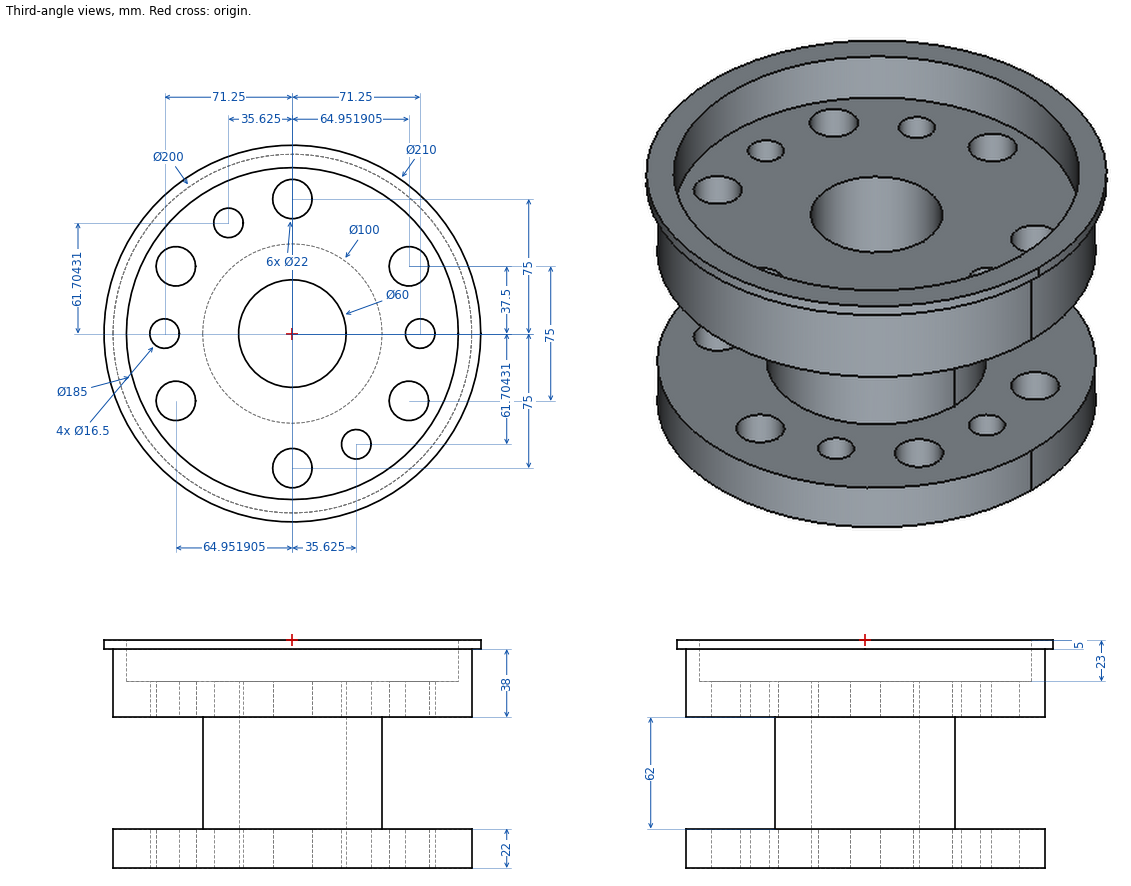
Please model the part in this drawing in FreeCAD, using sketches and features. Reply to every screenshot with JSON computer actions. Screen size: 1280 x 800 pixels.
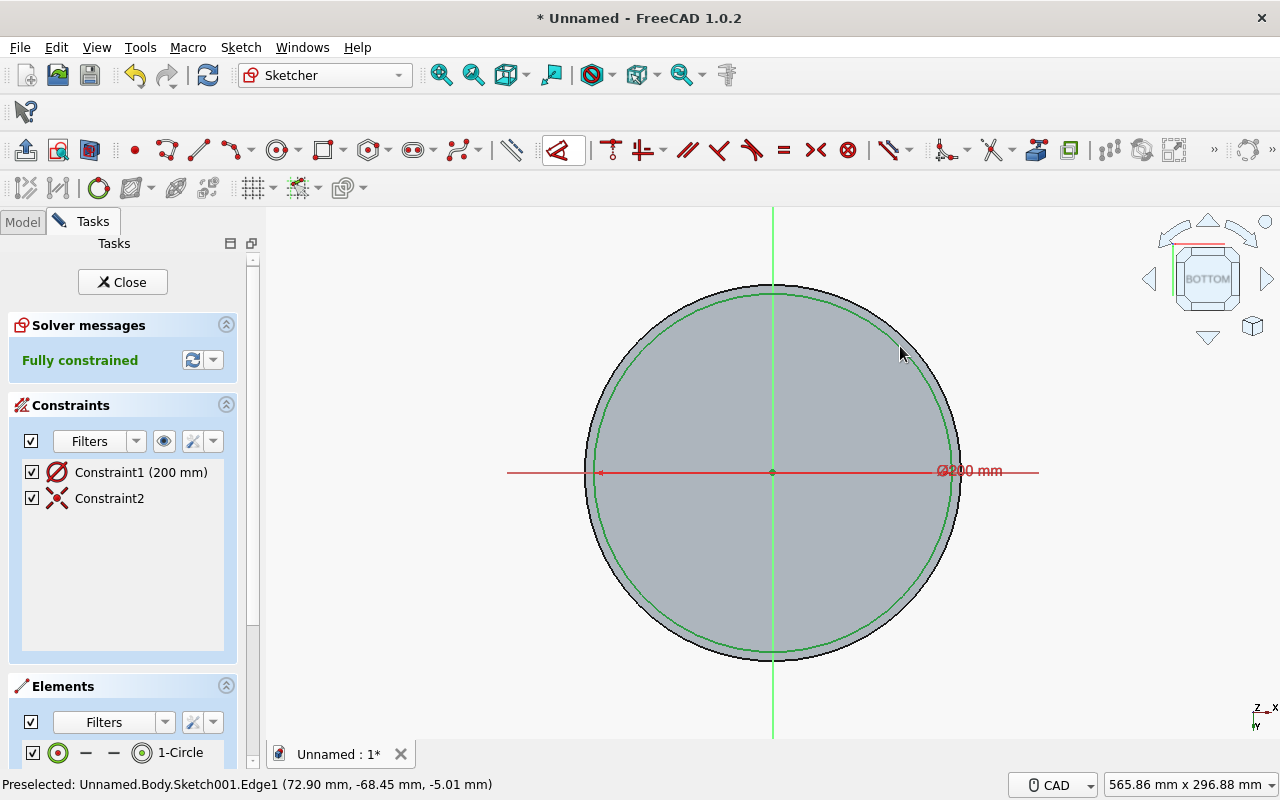
{"action": "left_click", "coordinate": [123, 282]}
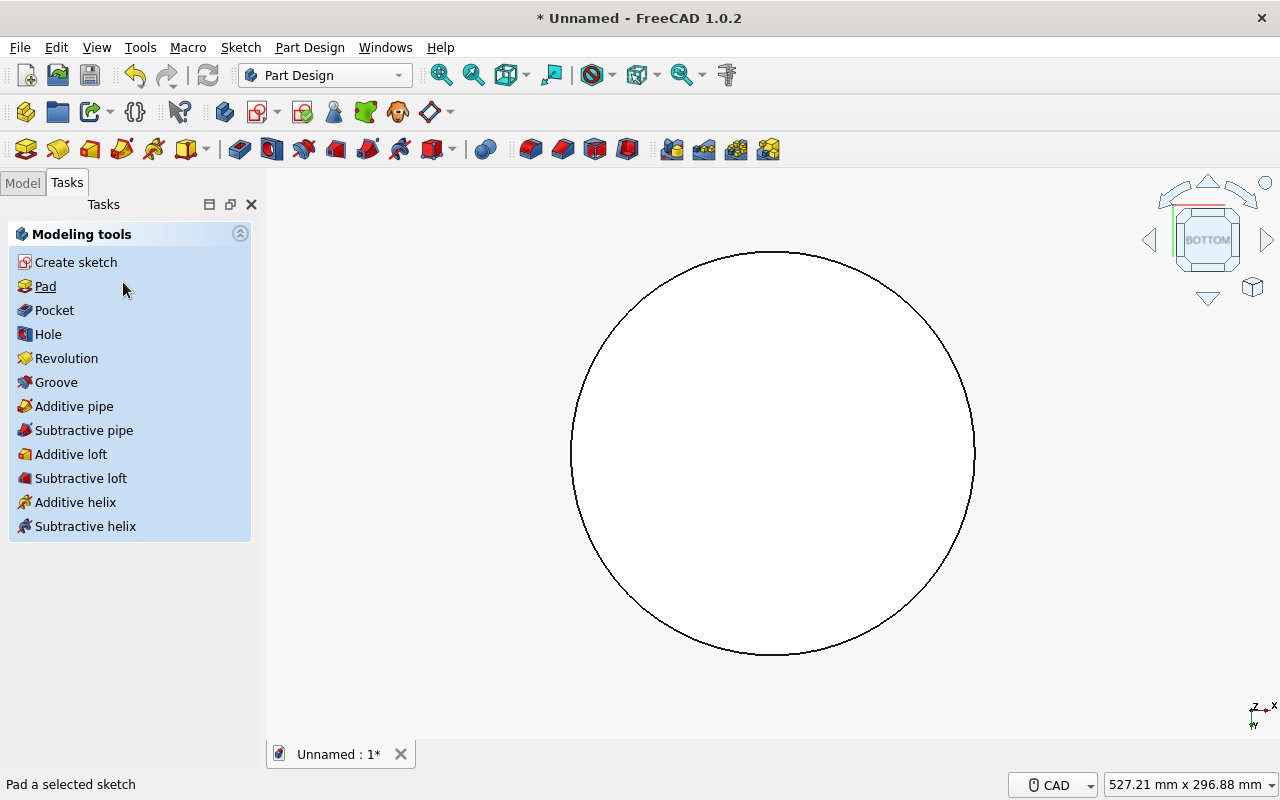
{"action": "left_click", "coordinate": [26, 150]}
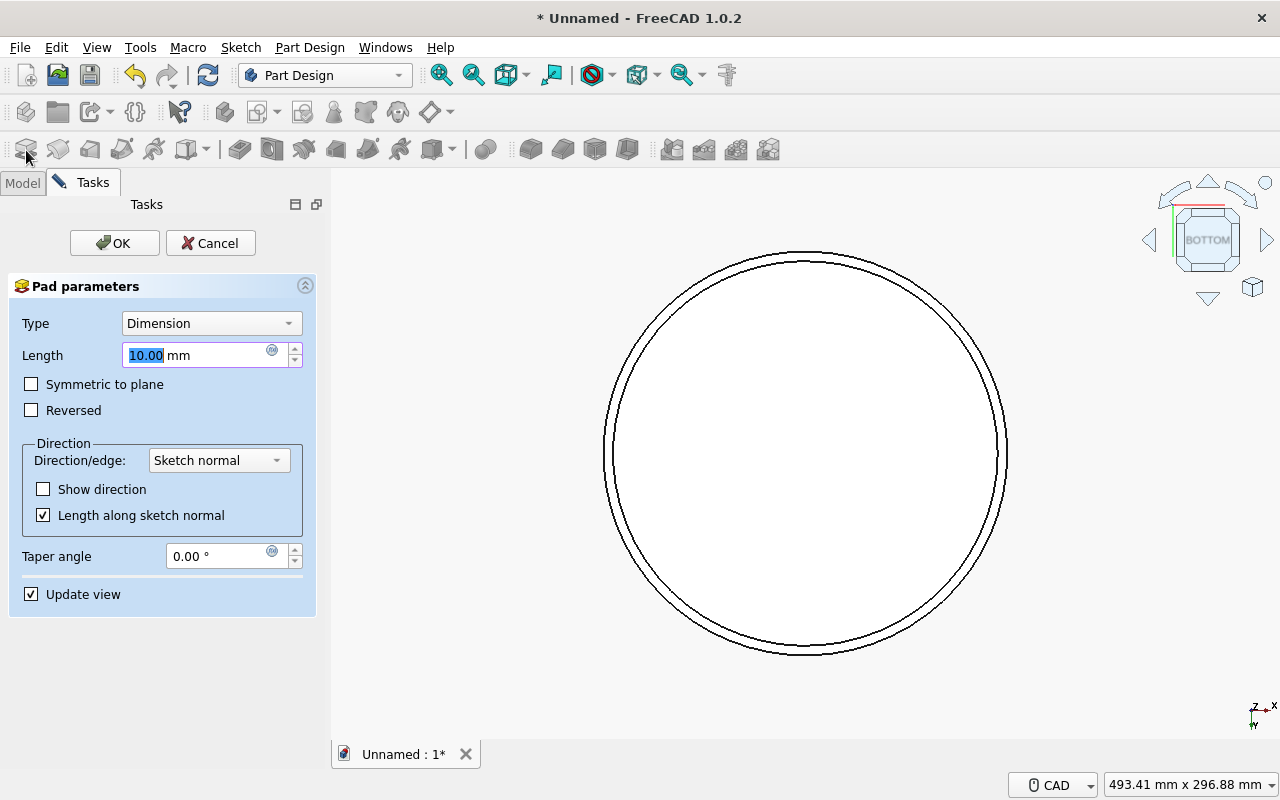
{"action": "type", "text": "38"}
{"action": "key", "text": "Tab"}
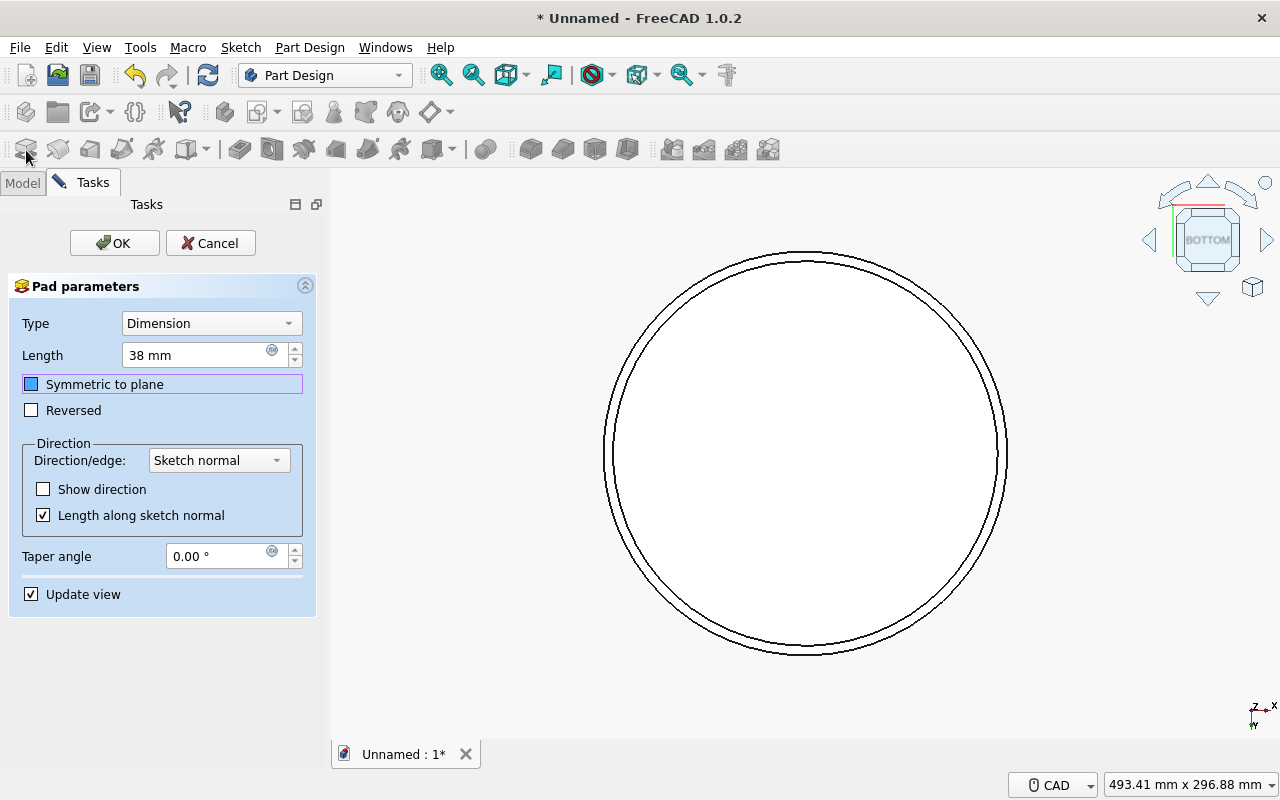
{"action": "left_click", "coordinate": [115, 243]}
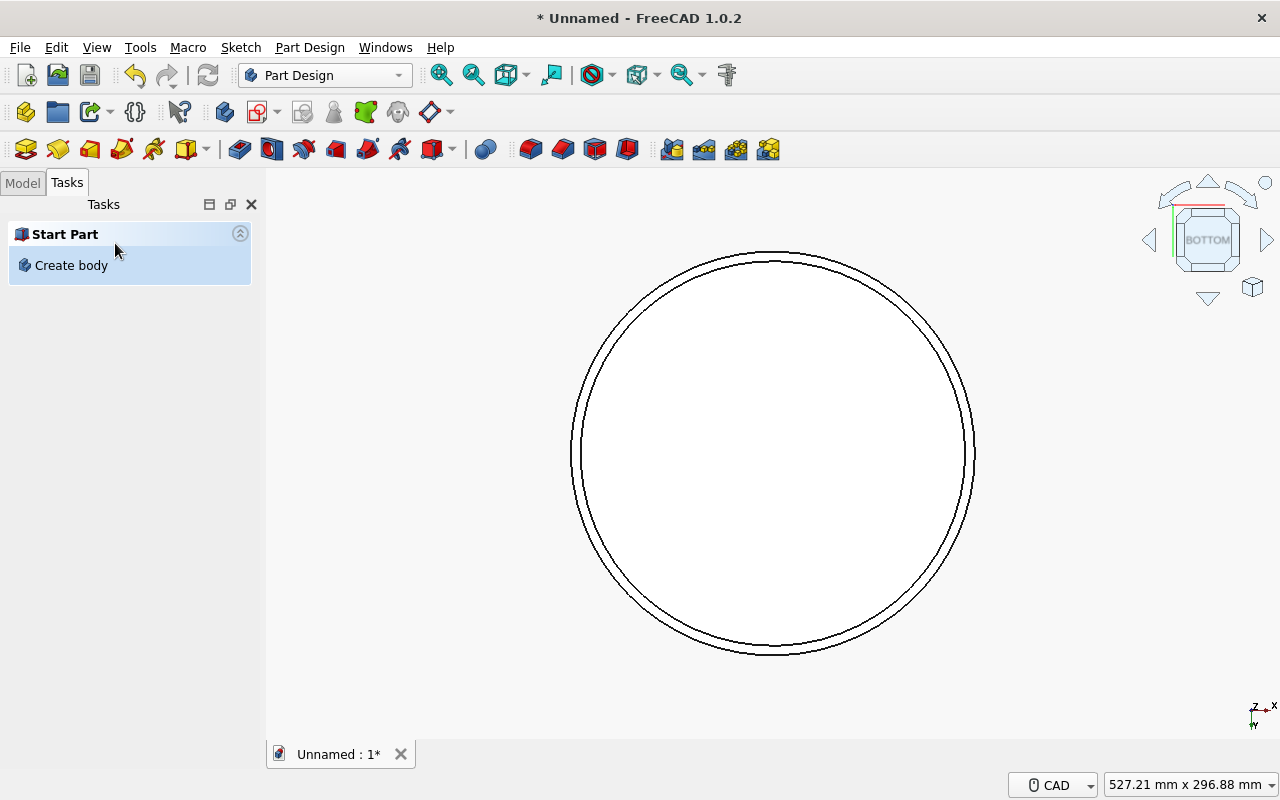
{"action": "left_click", "coordinate": [773, 453]}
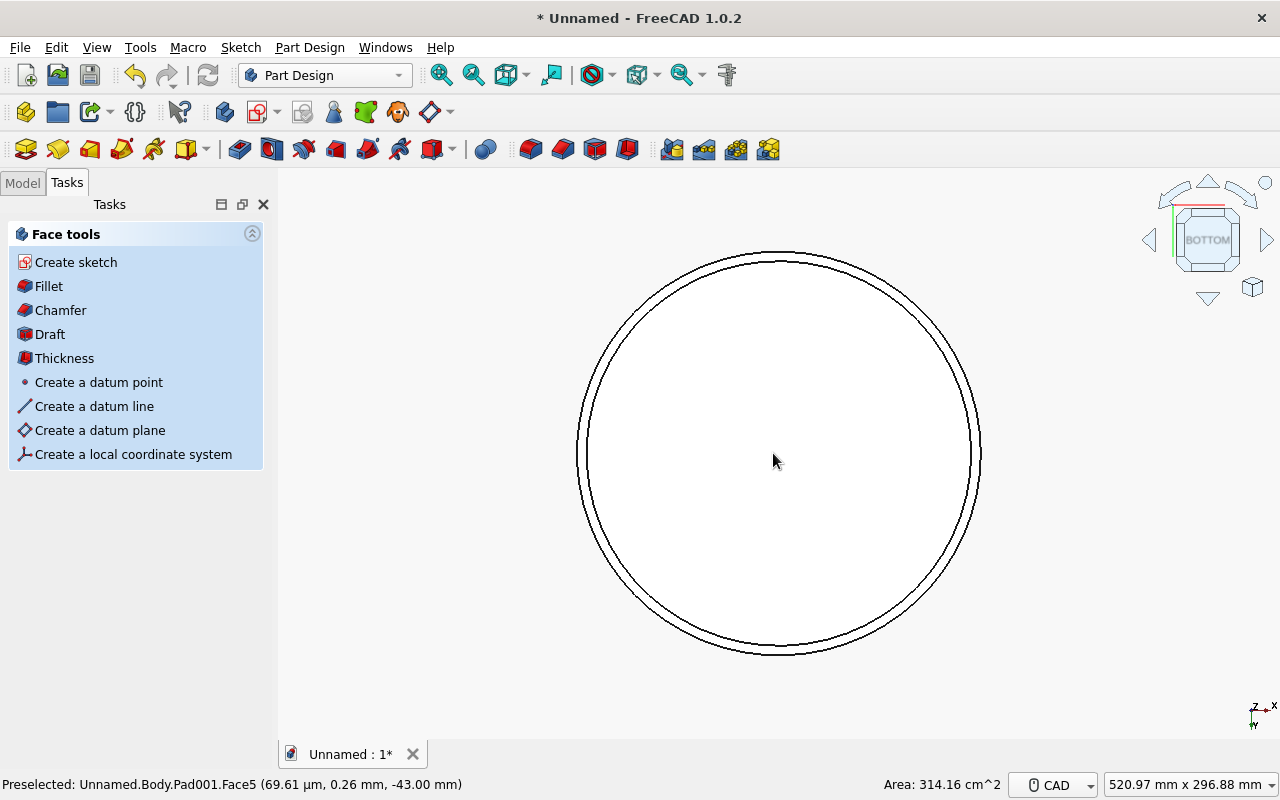
{"action": "left_click", "coordinate": [258, 112]}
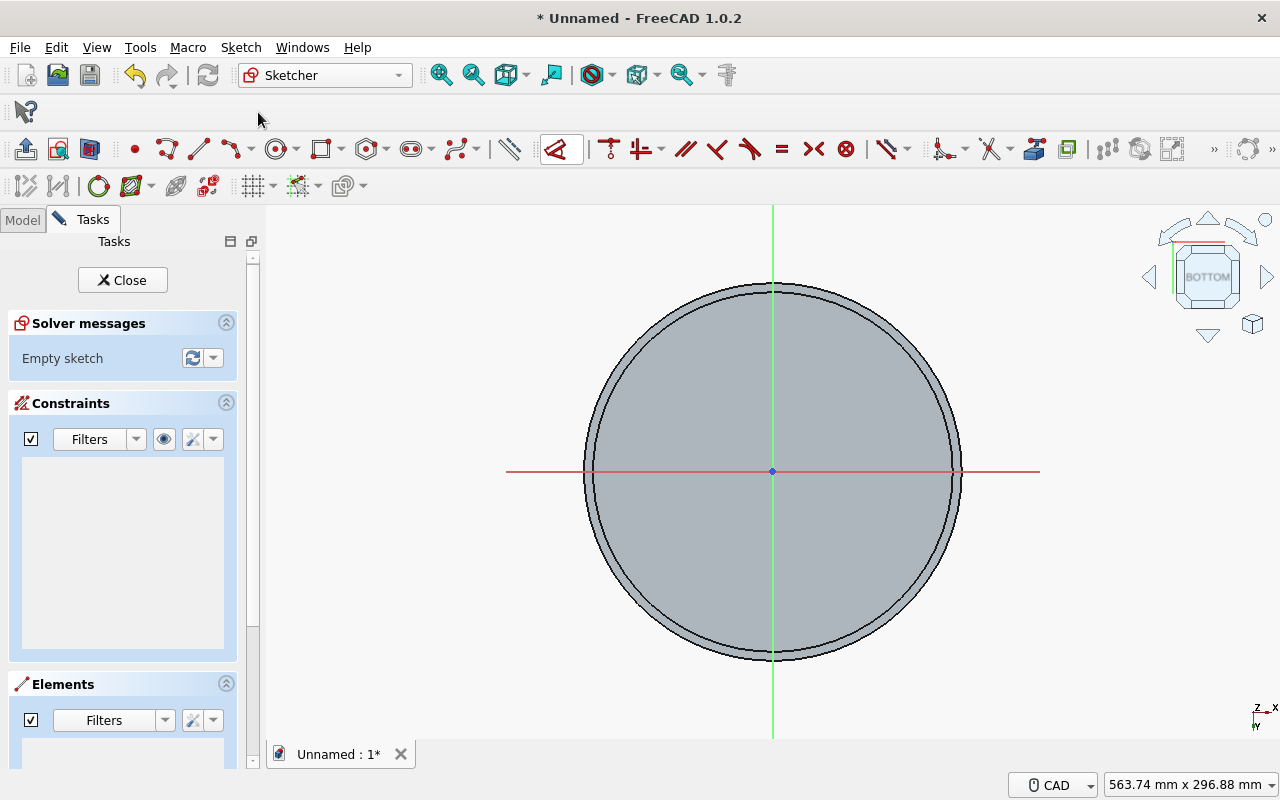
{"action": "scroll", "coordinate": [856, 472], "scroll_direction": "up", "scroll_amount": 3}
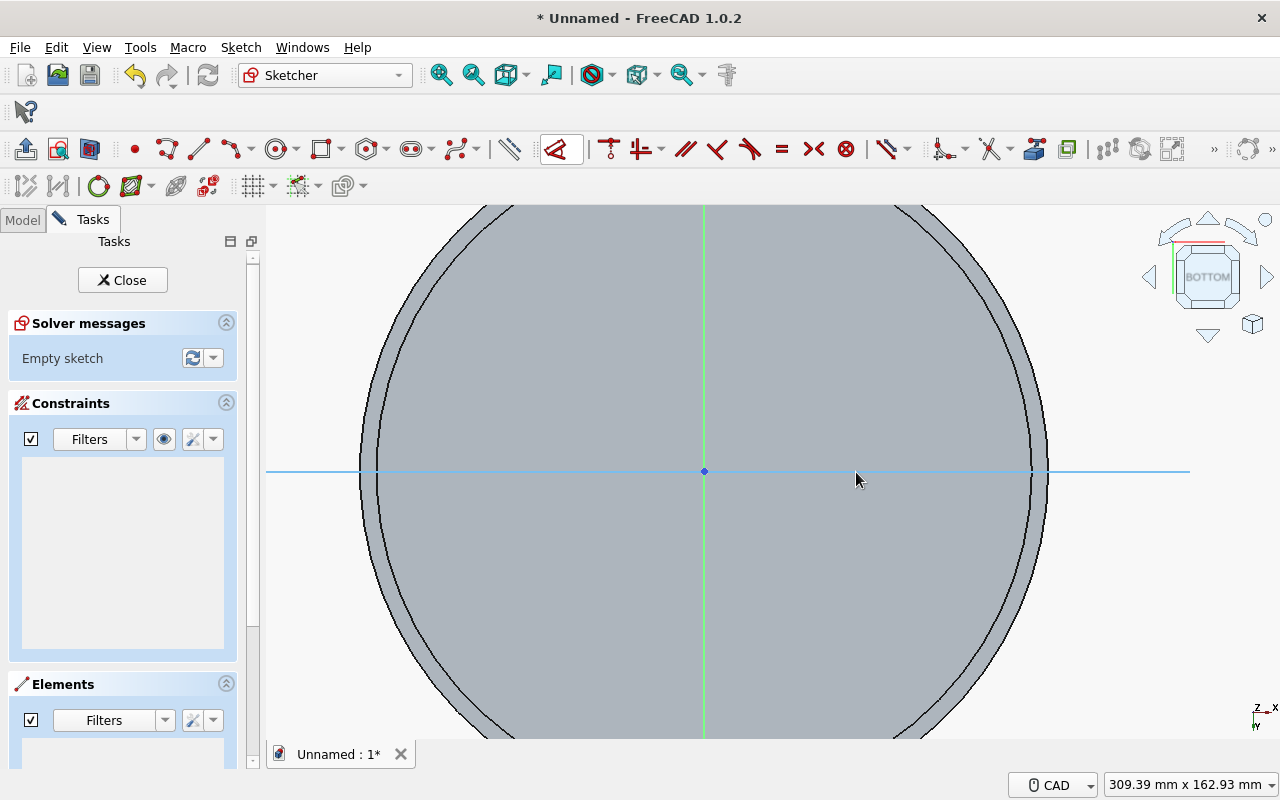
{"action": "left_click", "coordinate": [276, 150]}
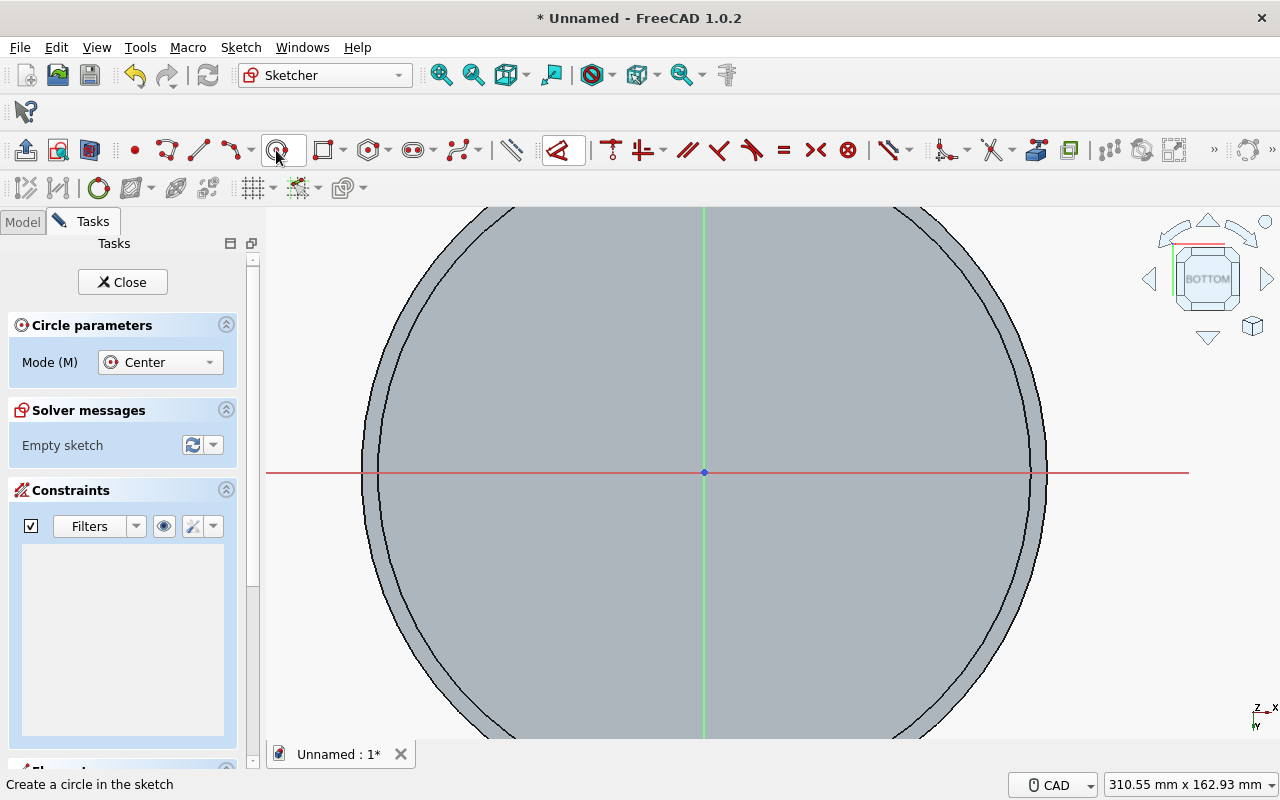
{"action": "left_click", "coordinate": [704, 473]}
{"action": "mouse_move", "coordinate": [820, 357]}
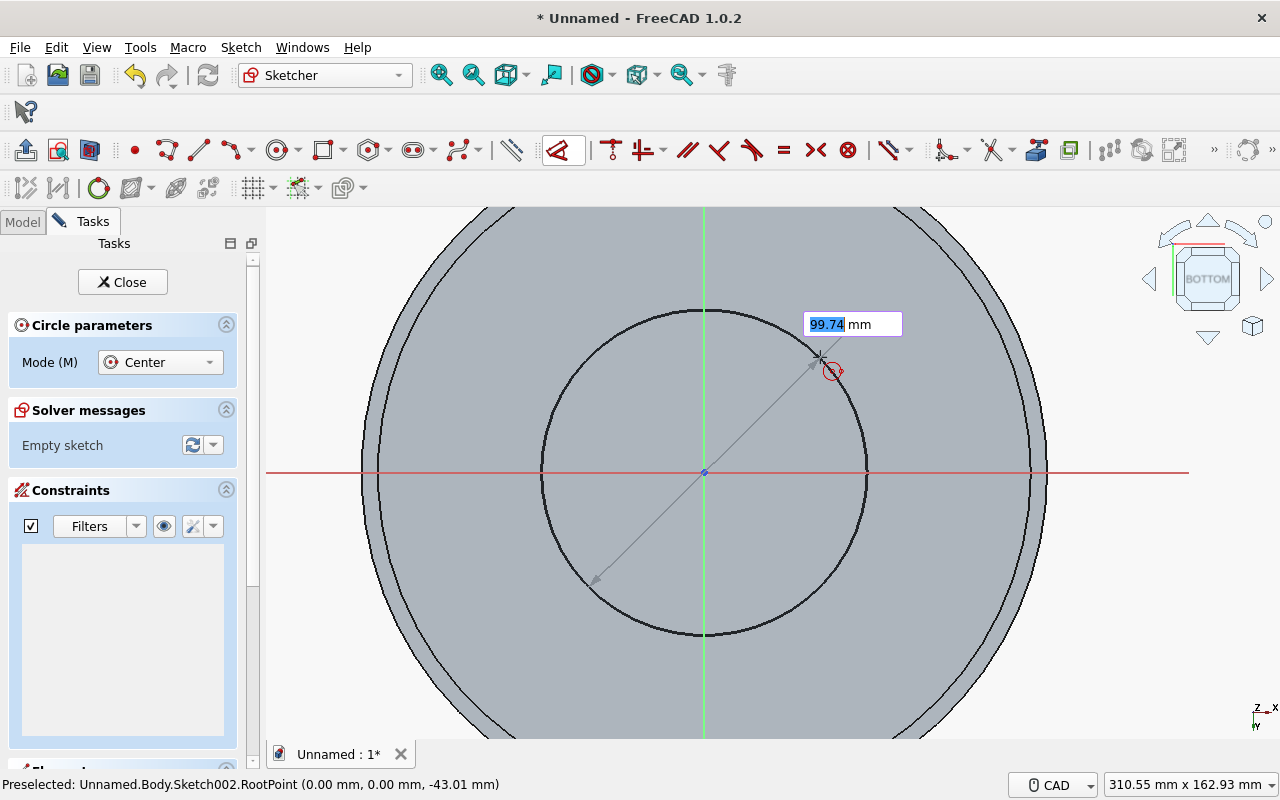
{"action": "type", "text": "100"}
{"action": "key", "text": "Return"}
{"action": "key", "text": "Escape"}